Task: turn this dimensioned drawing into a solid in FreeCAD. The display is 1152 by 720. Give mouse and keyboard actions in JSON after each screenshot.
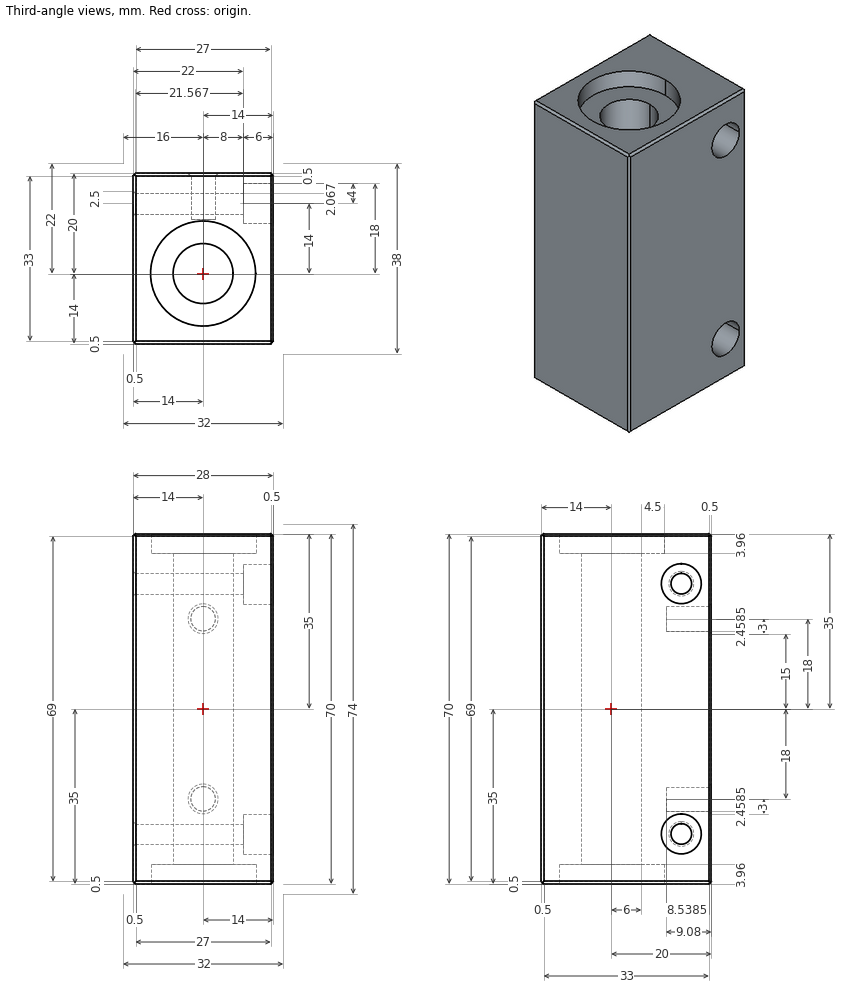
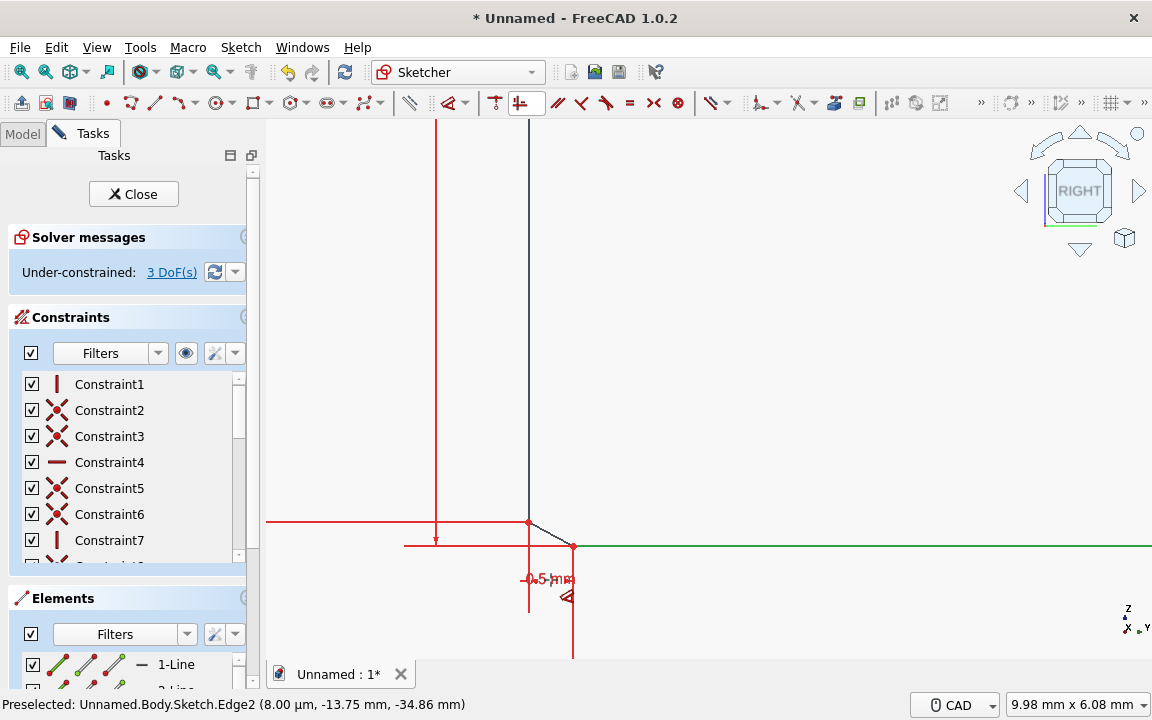
{"action": "left_click", "coordinate": [542, 529]}
{"action": "left_click", "coordinate": [495, 534]}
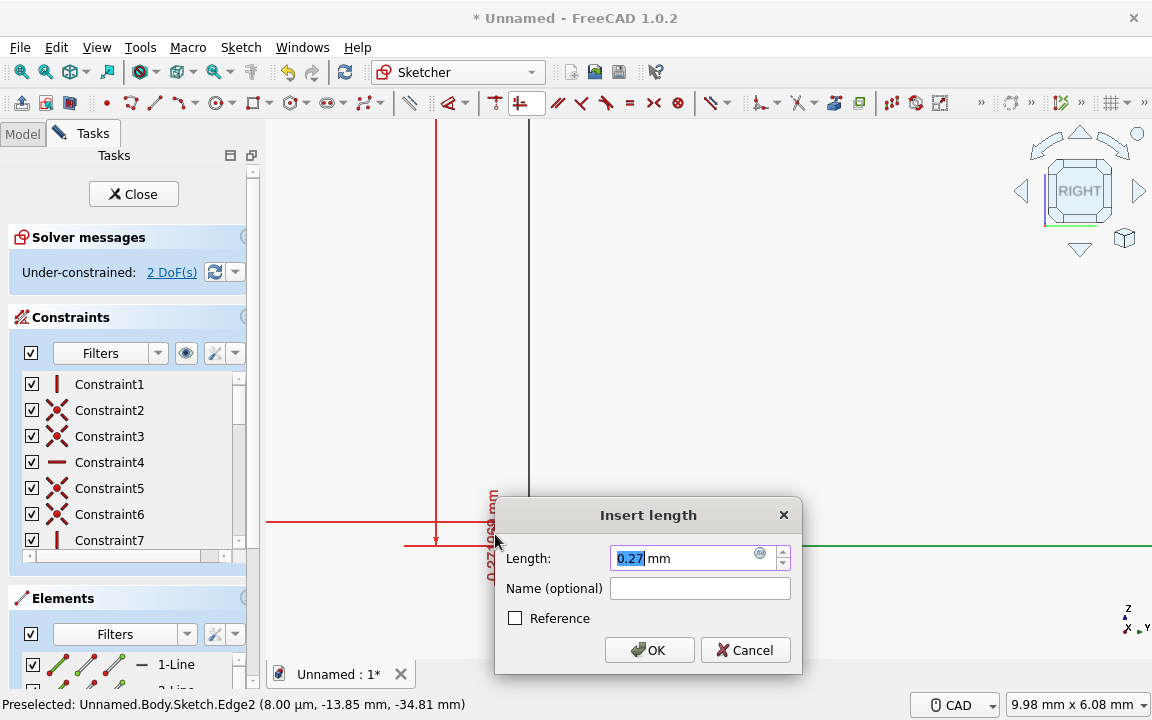
{"action": "type", "text": "0.5"}
{"action": "key", "text": "Return"}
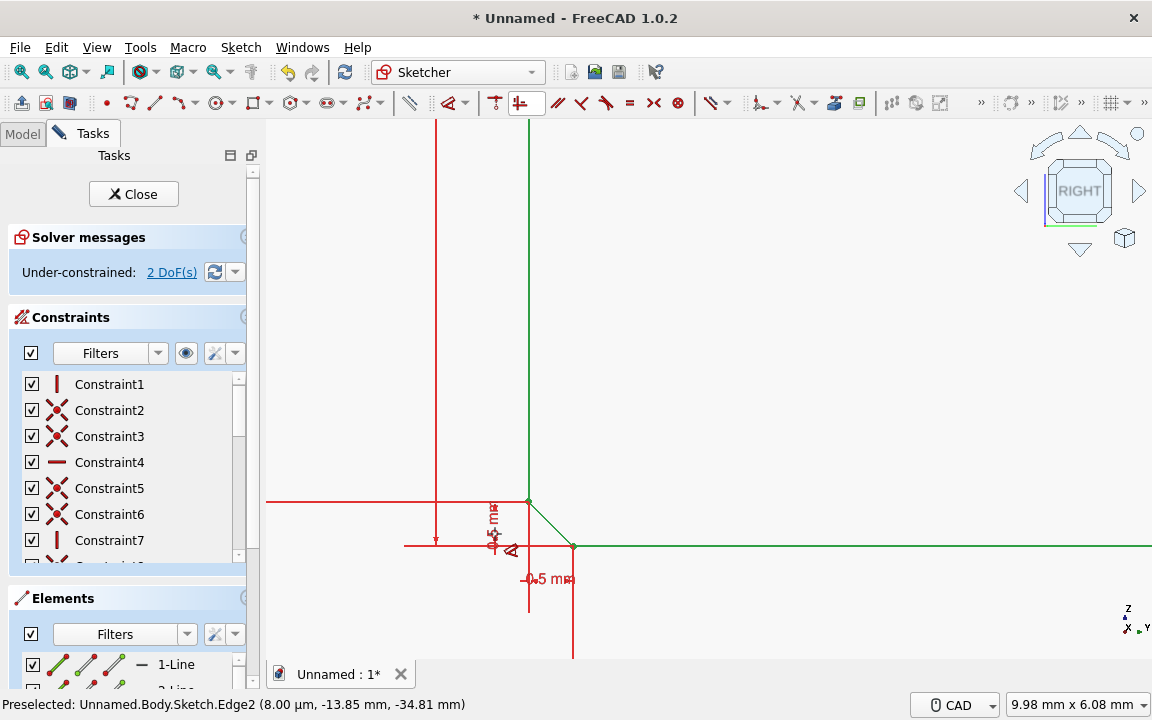
{"action": "scroll", "coordinate": [567, 544], "scroll_direction": "down", "scroll_amount": 15}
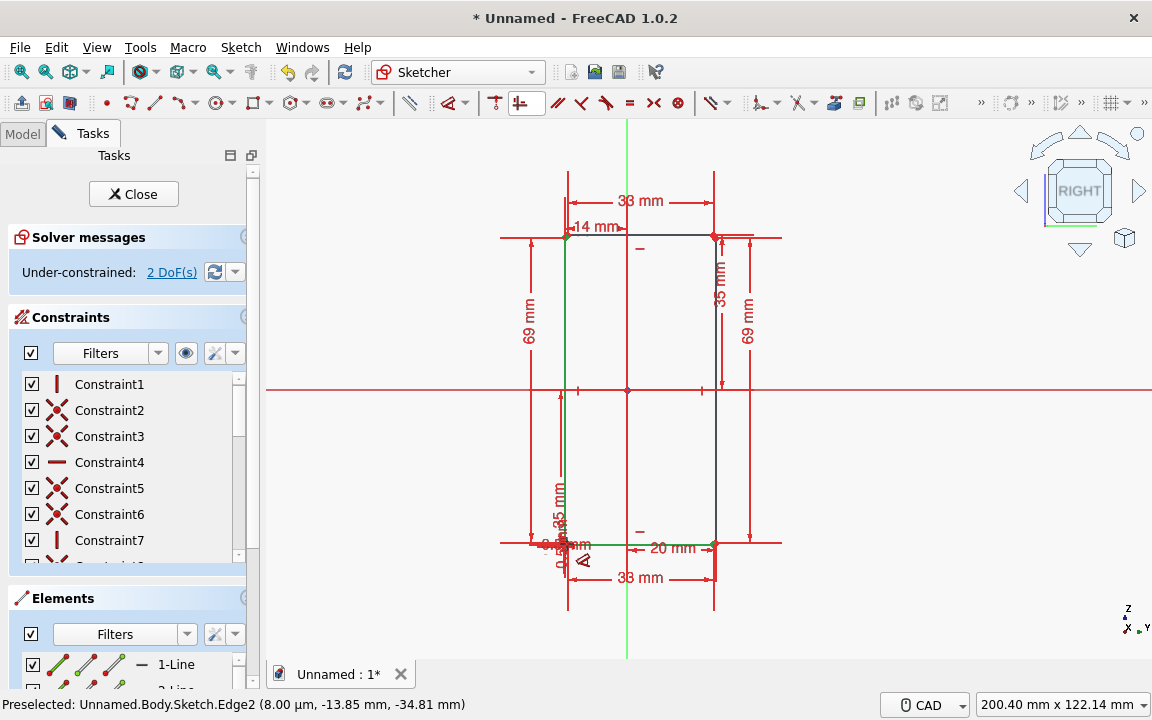
{"action": "scroll", "coordinate": [714, 544], "scroll_direction": "up", "scroll_amount": 15}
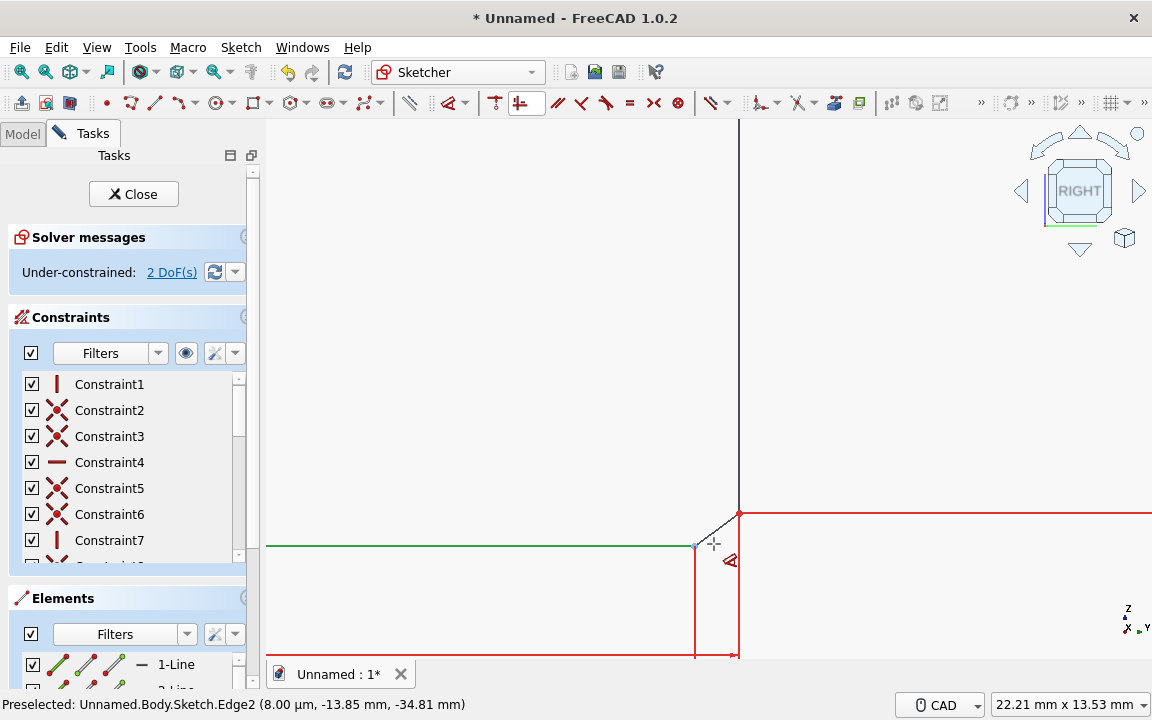
{"action": "left_click", "coordinate": [708, 536]}
{"action": "left_click", "coordinate": [773, 530]}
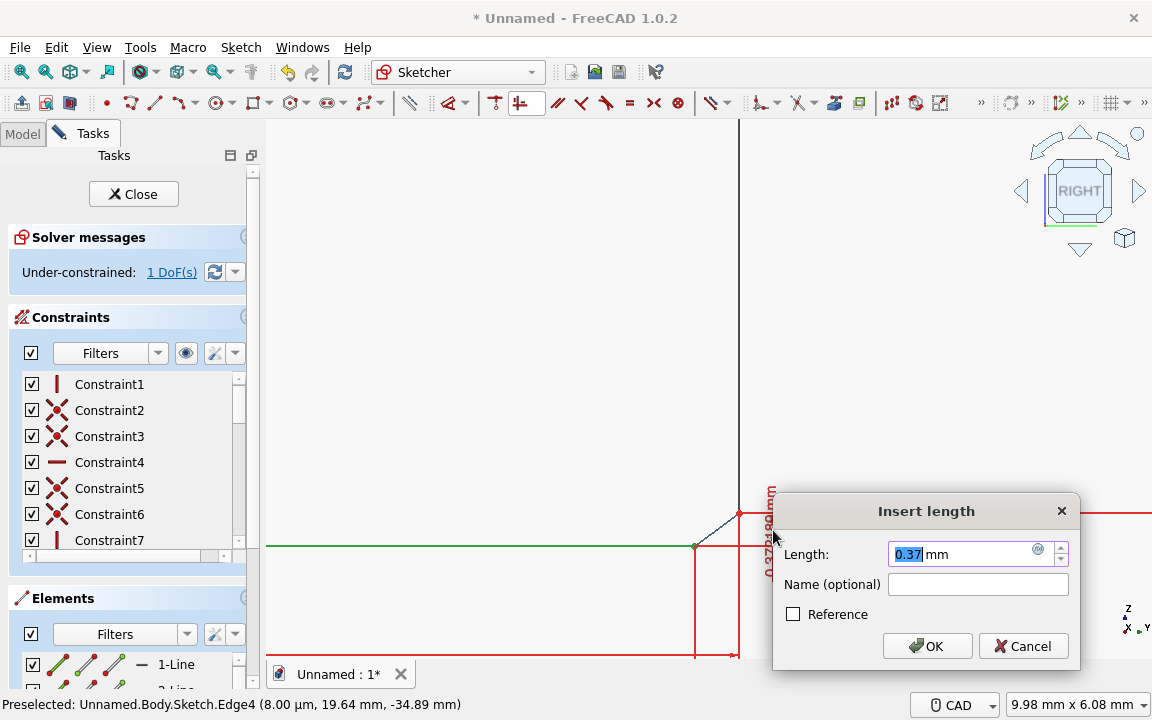
{"action": "type", "text": "0.5"}
{"action": "key", "text": "Return"}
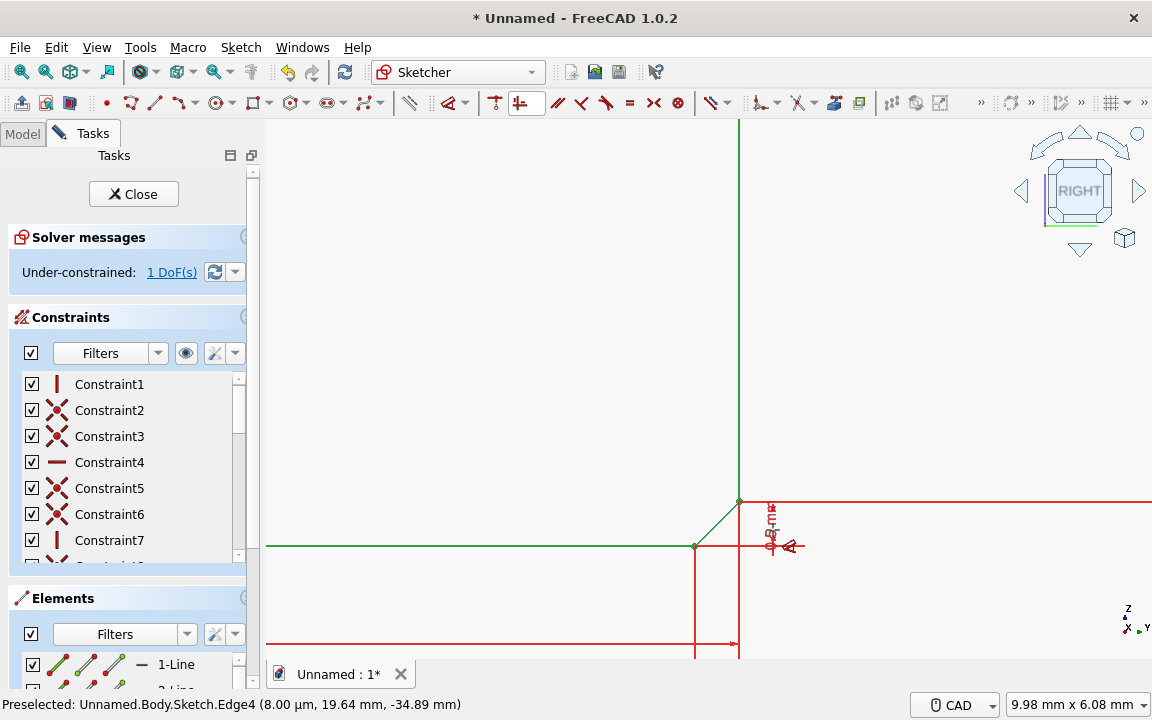
{"action": "scroll", "coordinate": [714, 544], "scroll_direction": "down", "scroll_amount": 15}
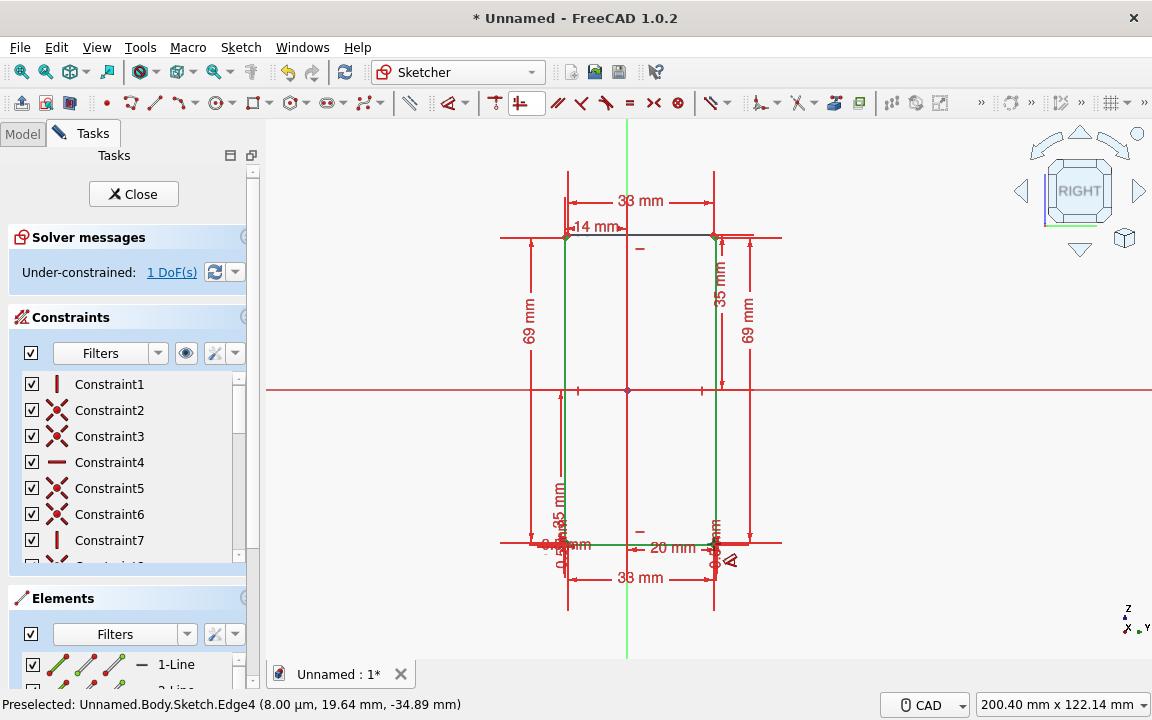
{"action": "scroll", "coordinate": [715, 237], "scroll_direction": "up", "scroll_amount": 15}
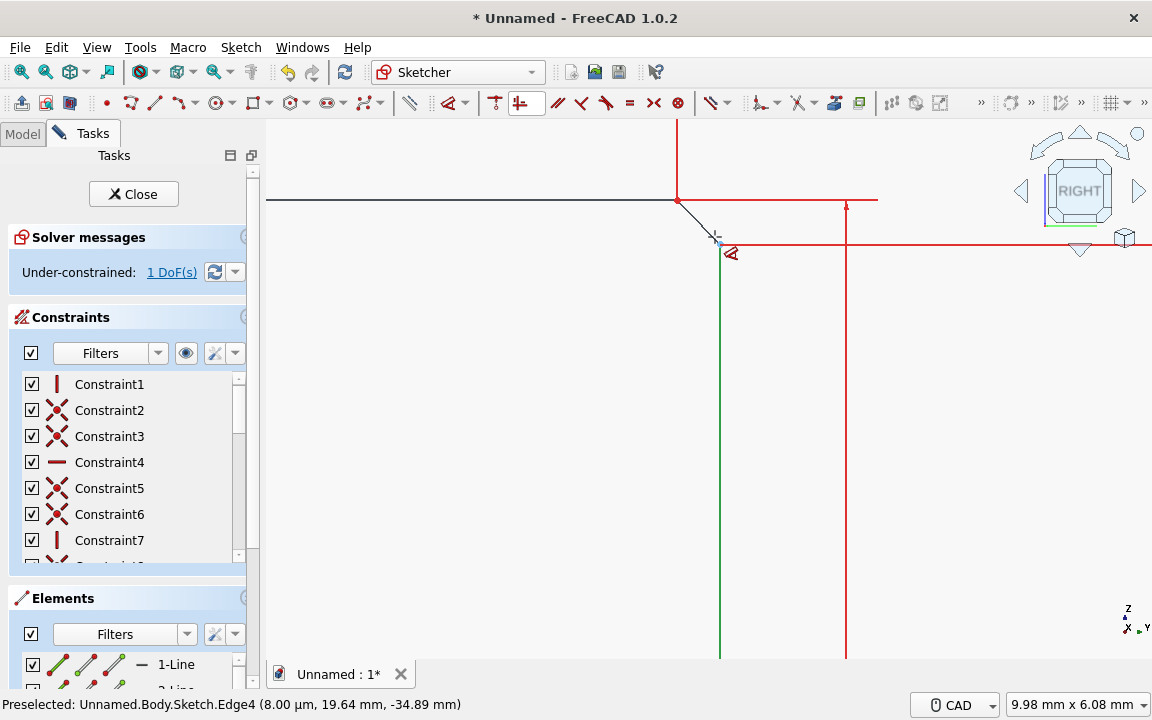
{"action": "left_click", "coordinate": [707, 231]}
{"action": "left_click", "coordinate": [699, 166]}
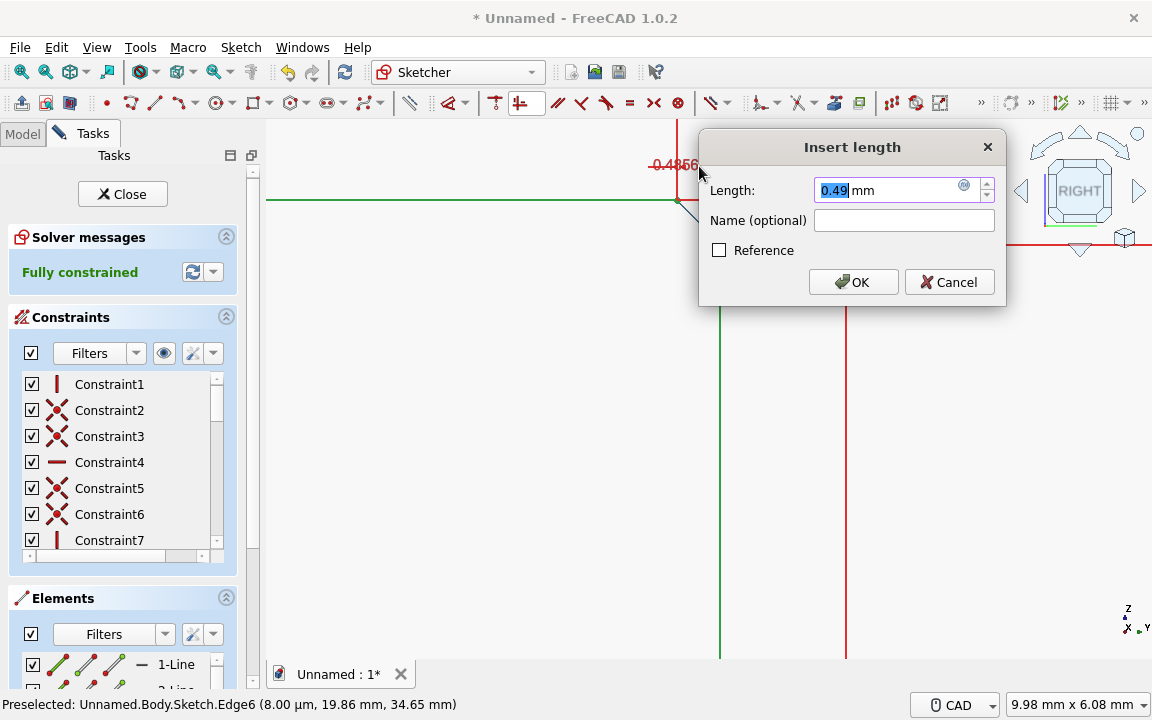
{"action": "type", "text": "0.5"}
{"action": "key", "text": "Return"}
{"action": "key", "text": "Escape"}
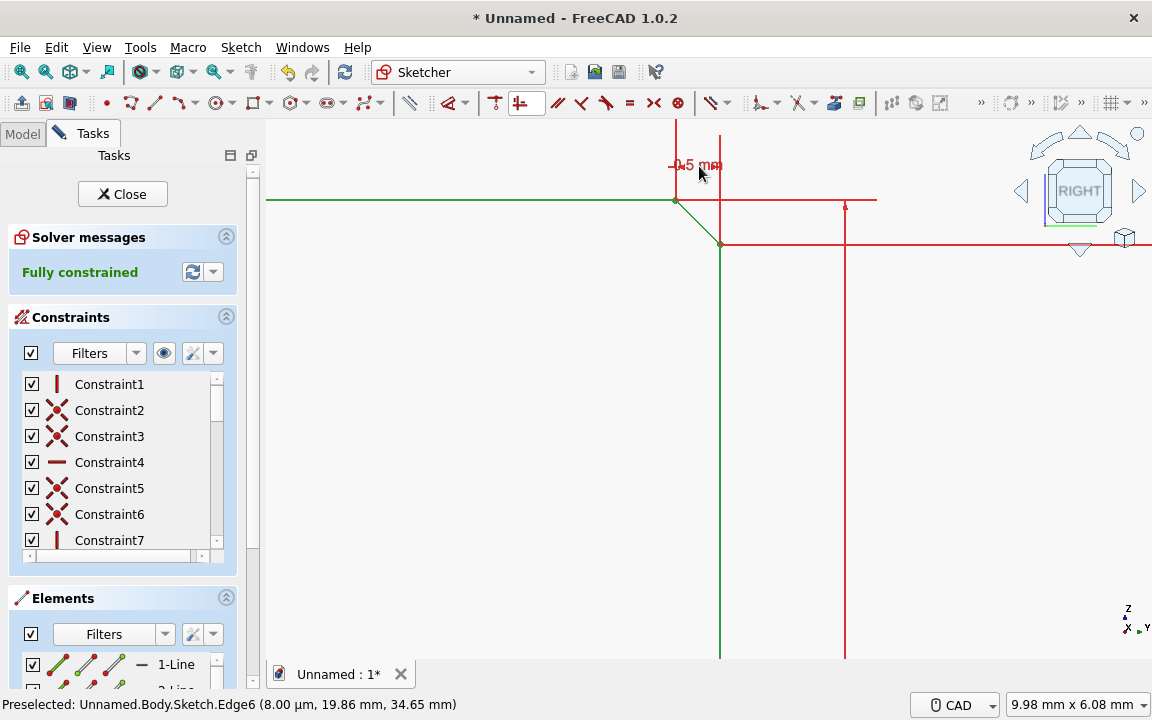
{"action": "left_click", "coordinate": [123, 194]}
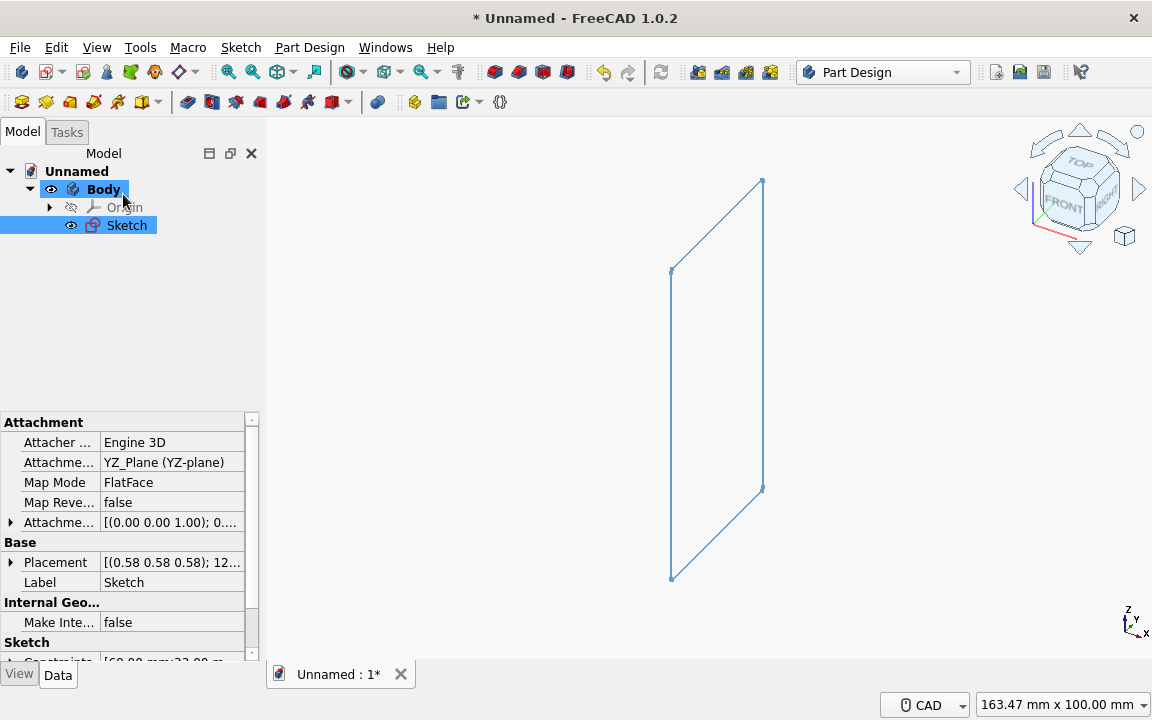
{"action": "left_click", "coordinate": [22, 102]}